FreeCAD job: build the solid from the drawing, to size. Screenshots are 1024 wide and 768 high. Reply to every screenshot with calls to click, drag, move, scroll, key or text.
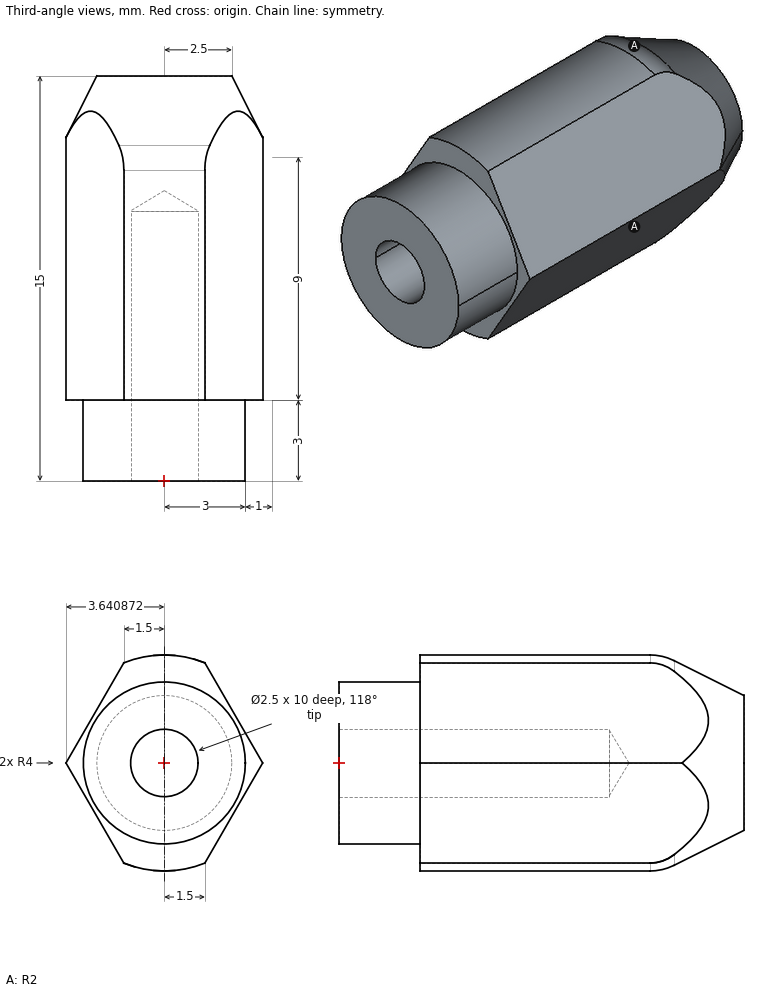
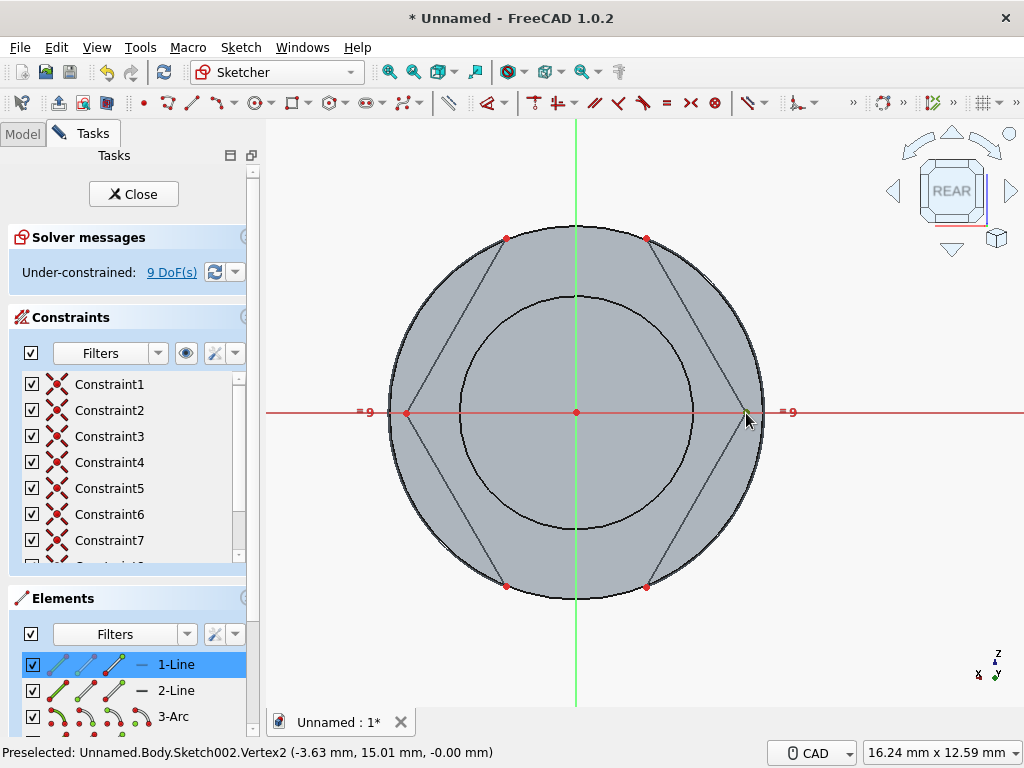
click(406, 414)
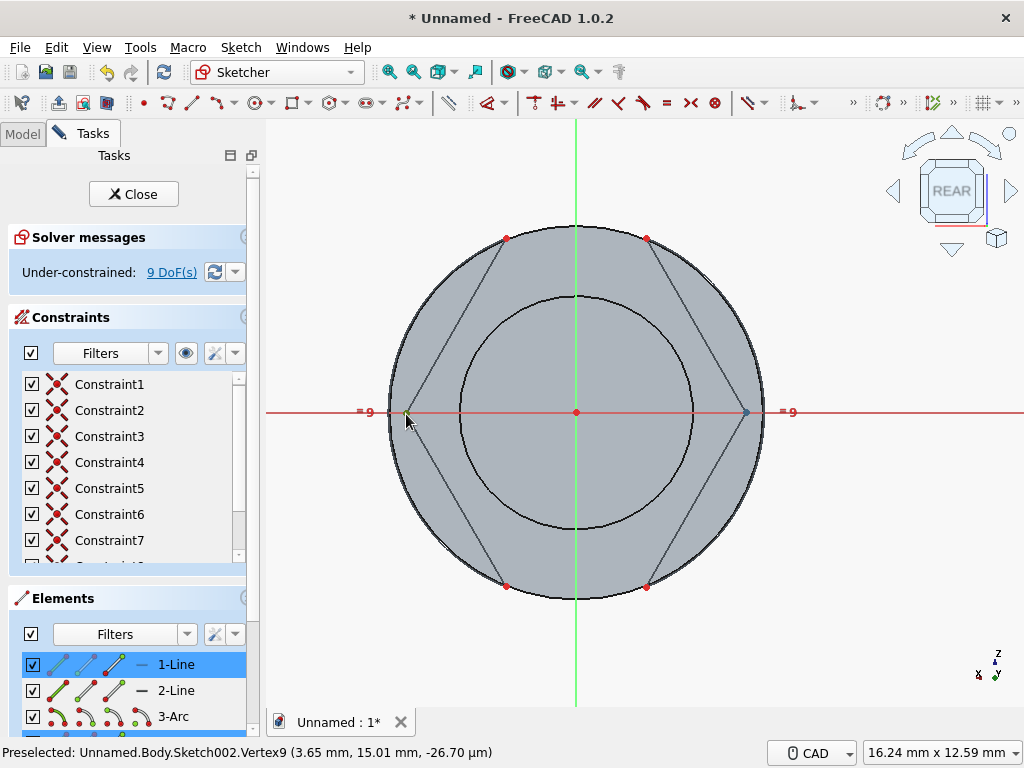
click(576, 641)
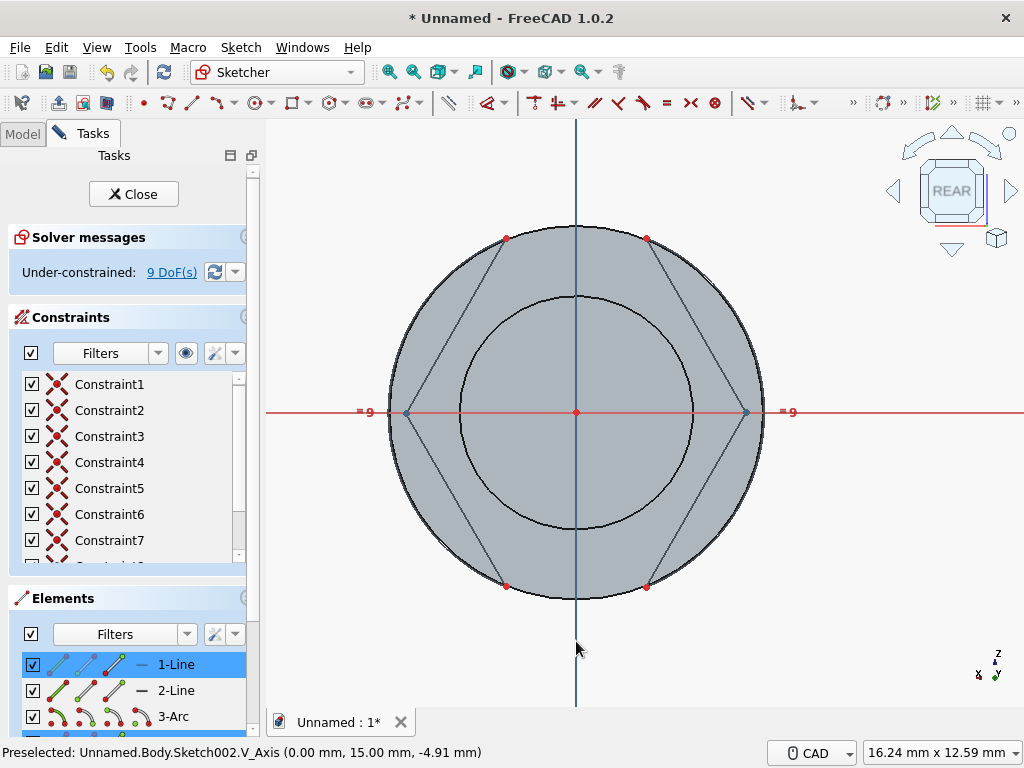
click(692, 104)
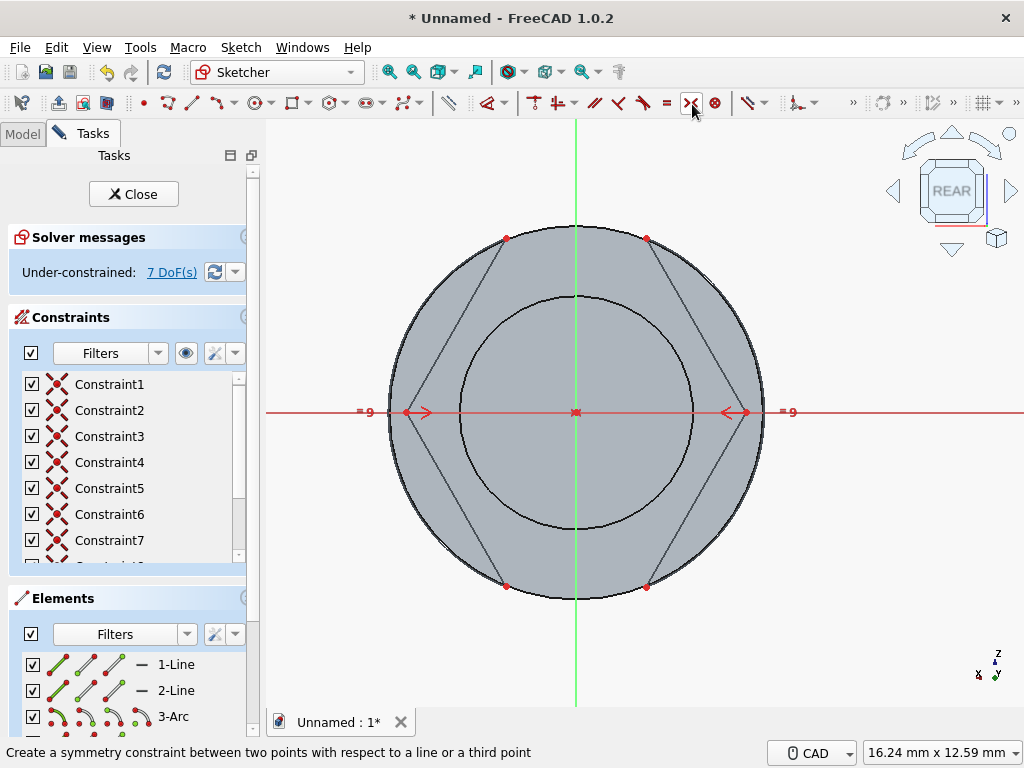
click(488, 104)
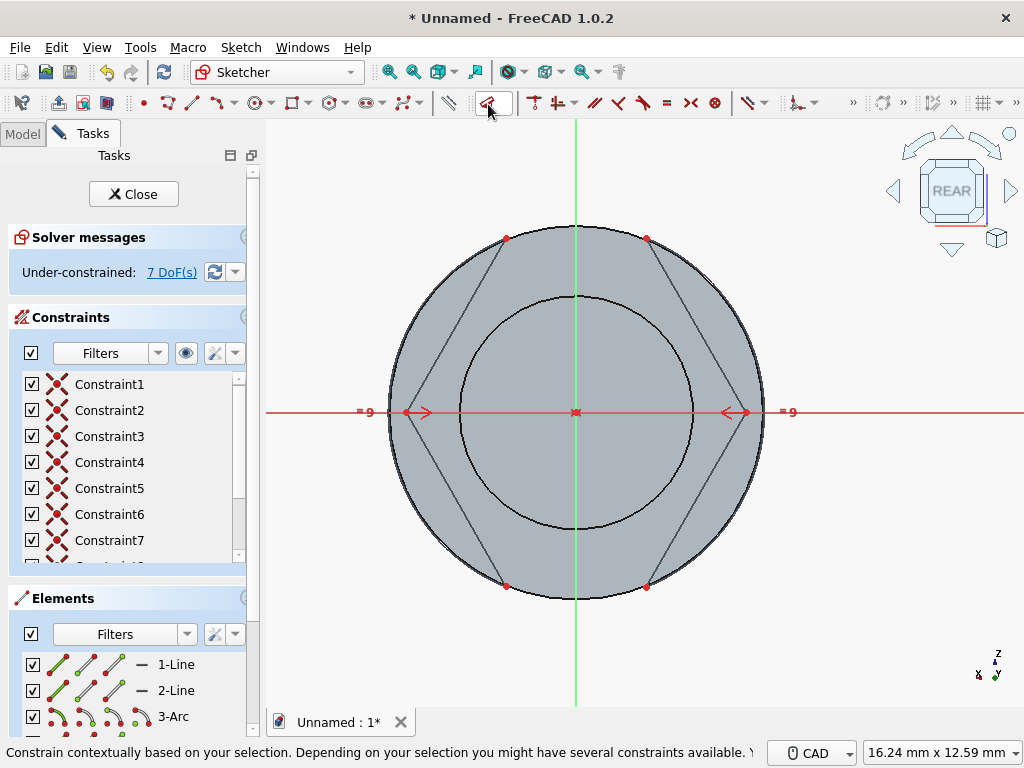
click(743, 499)
click(771, 514)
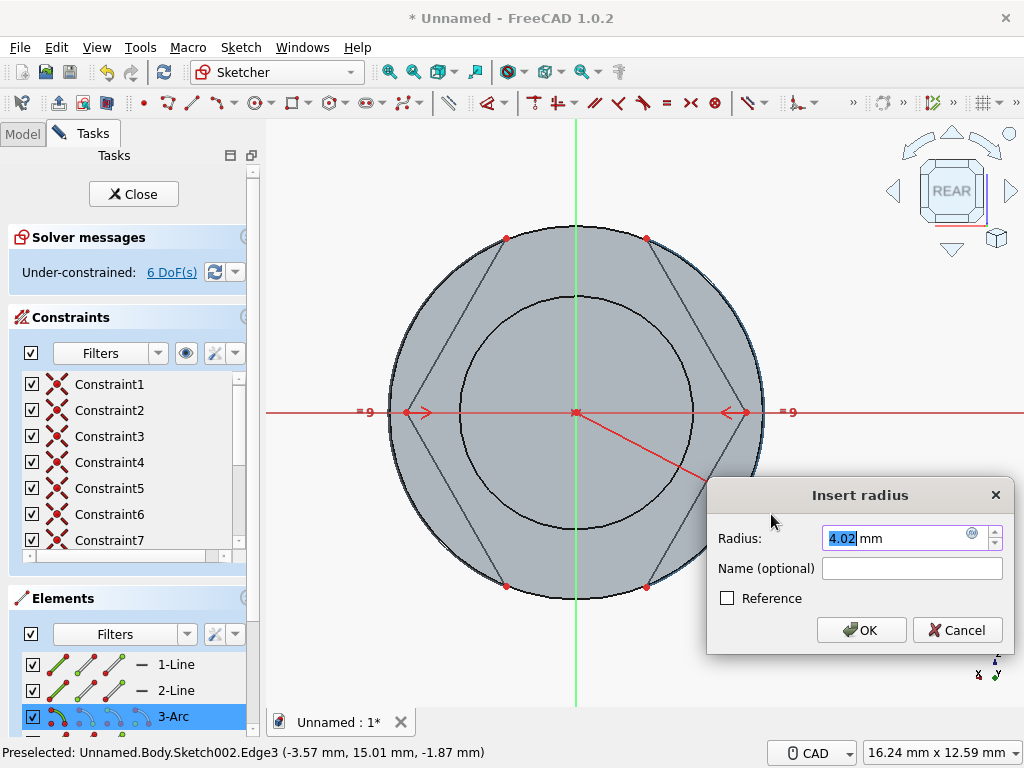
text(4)
key(Return)
key(Escape)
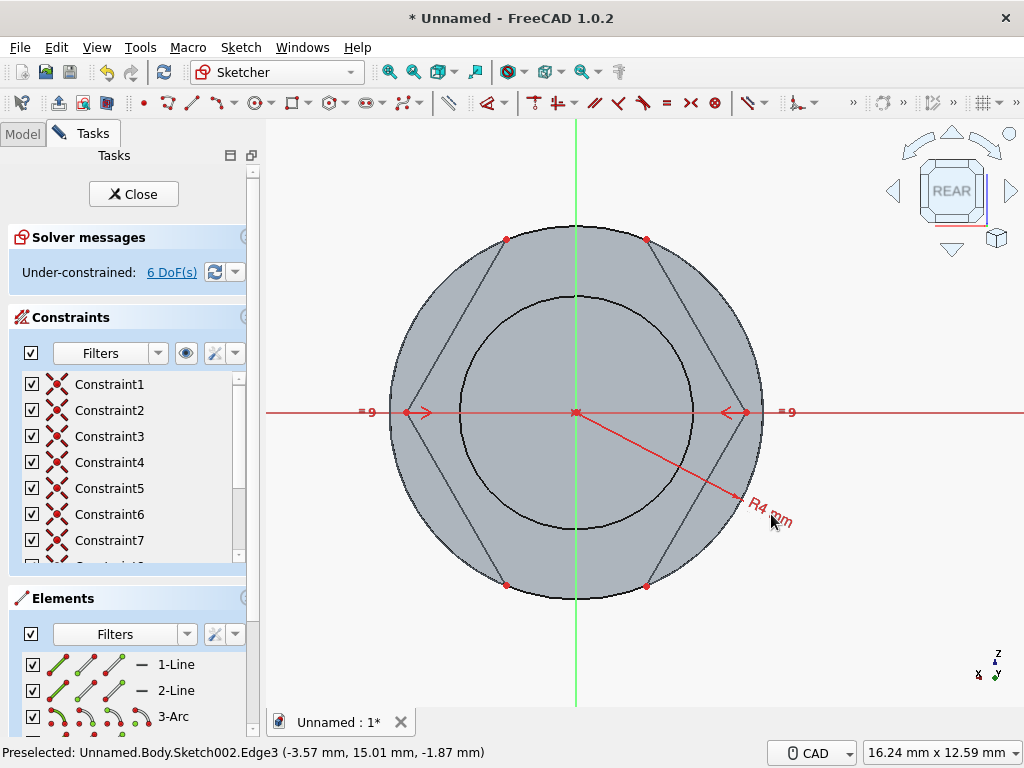
click(746, 413)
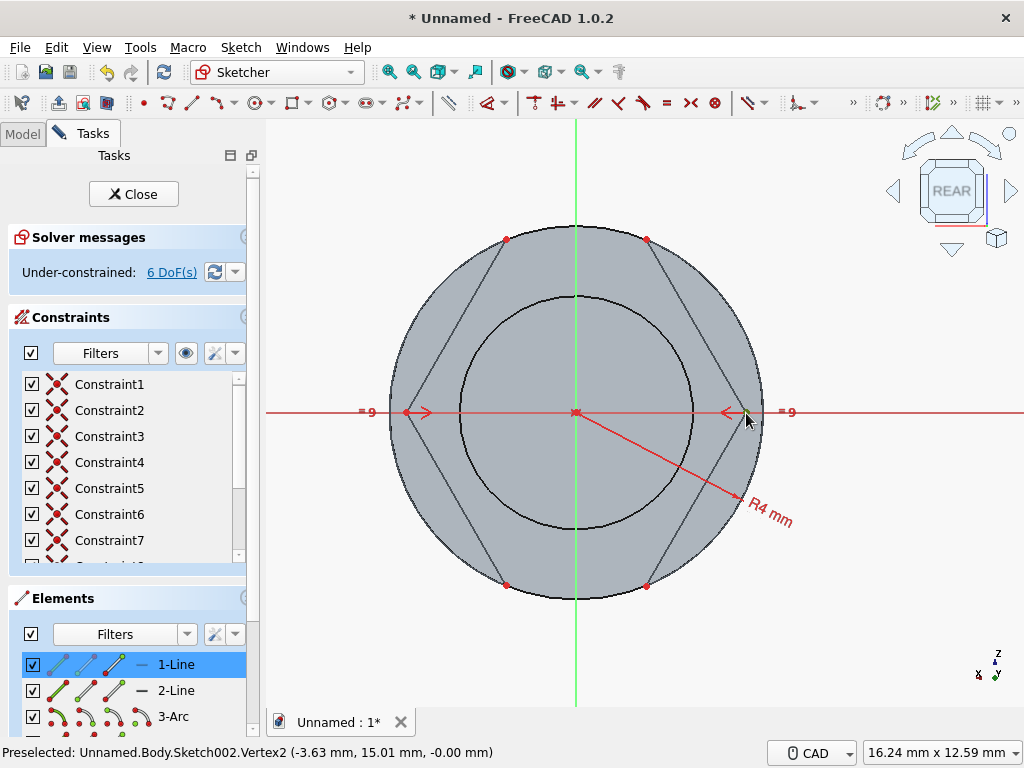
click(334, 413)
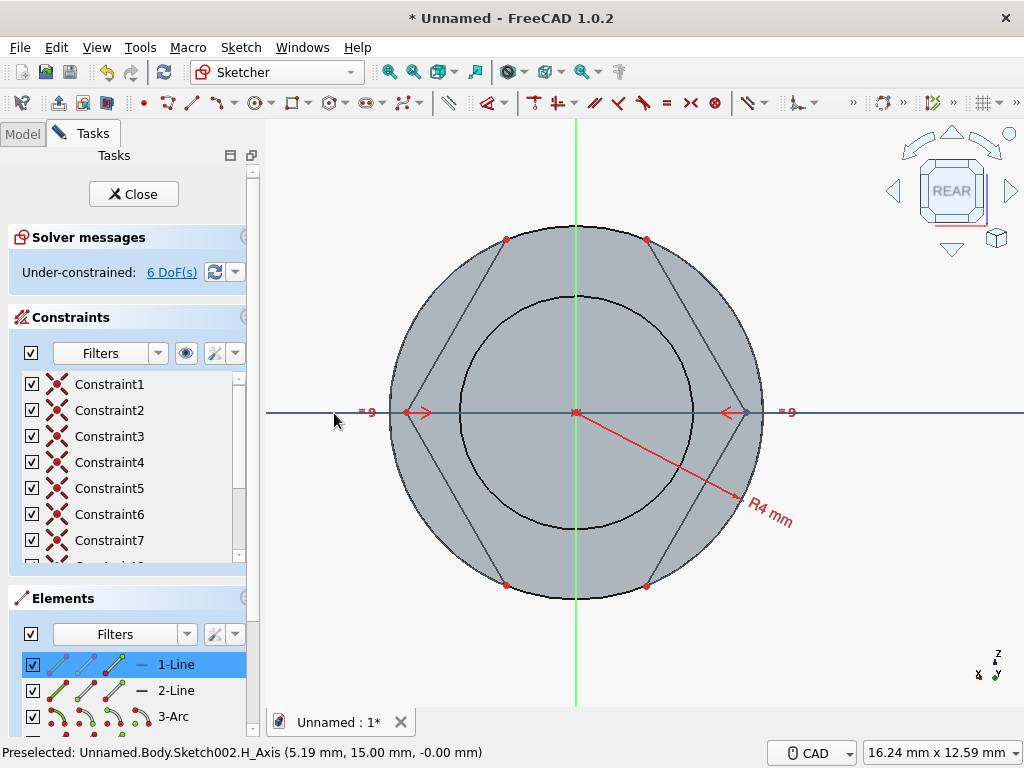
click(534, 104)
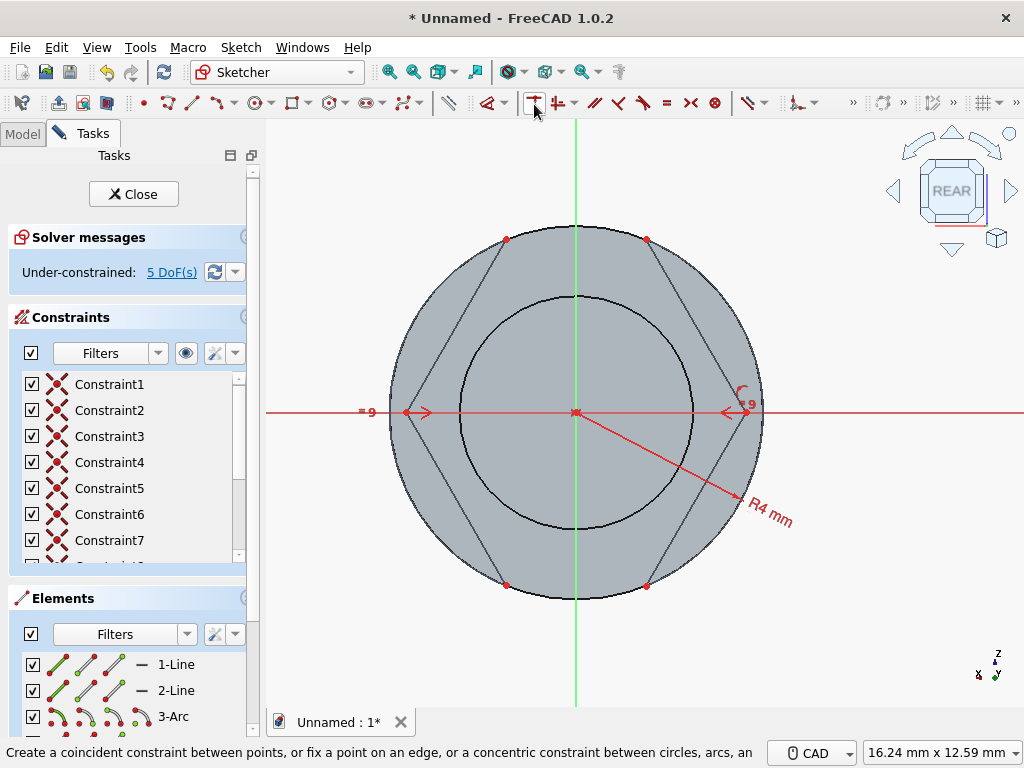
click(488, 104)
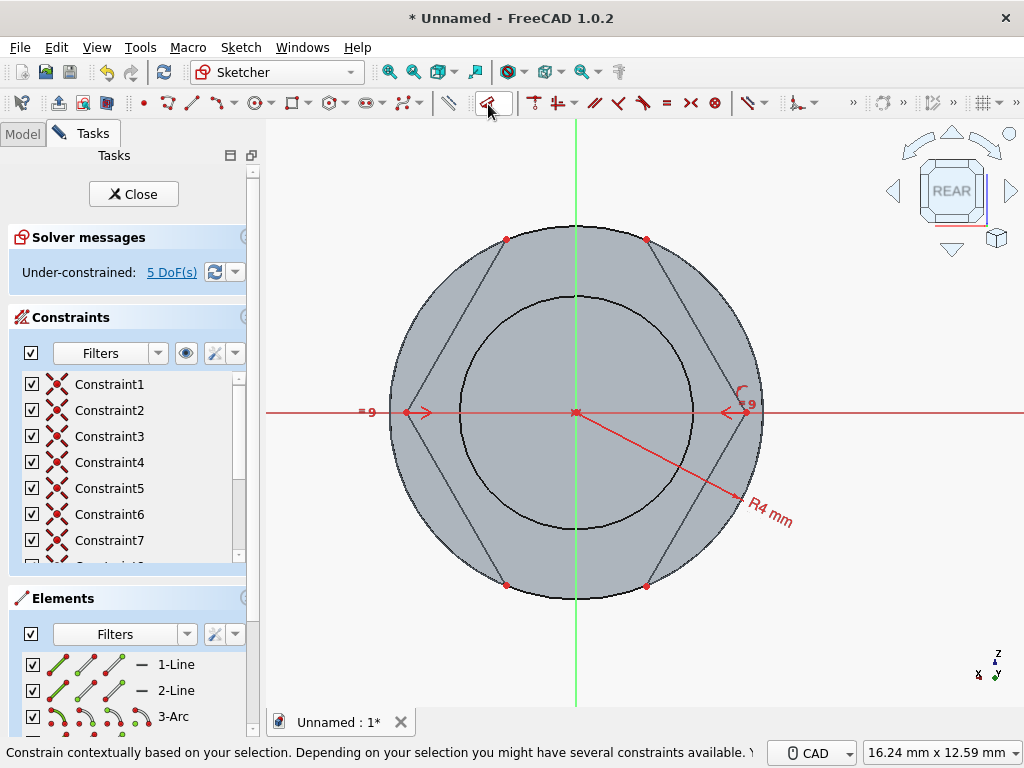
click(646, 239)
click(611, 205)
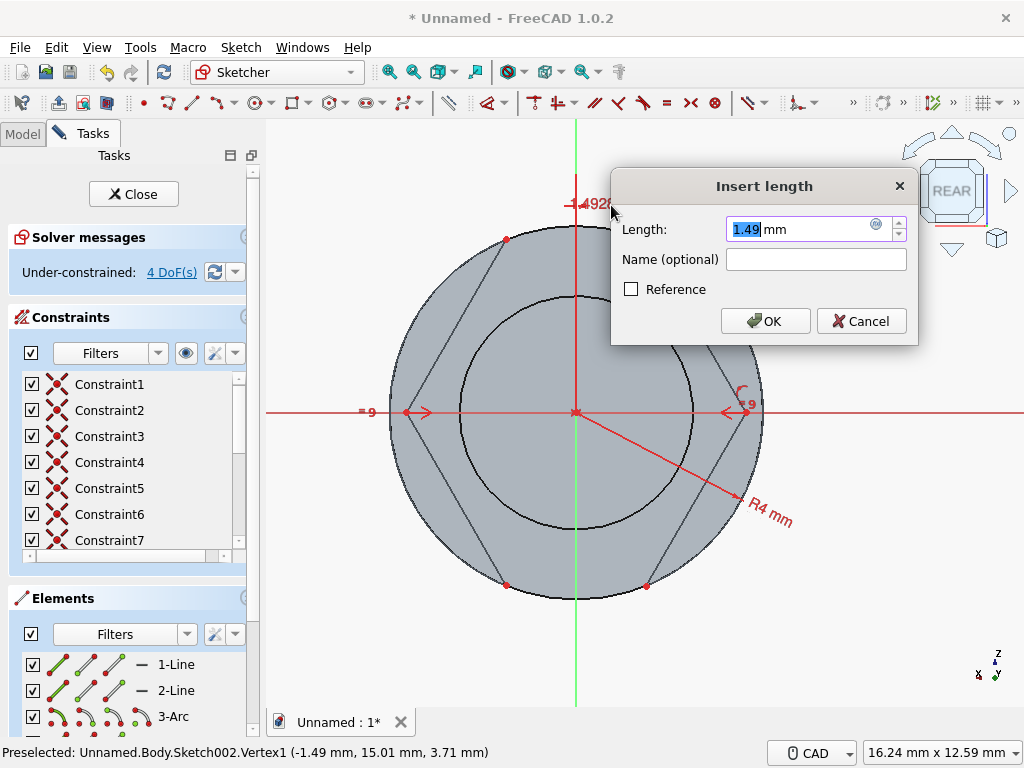
text(1.5)
key(Return)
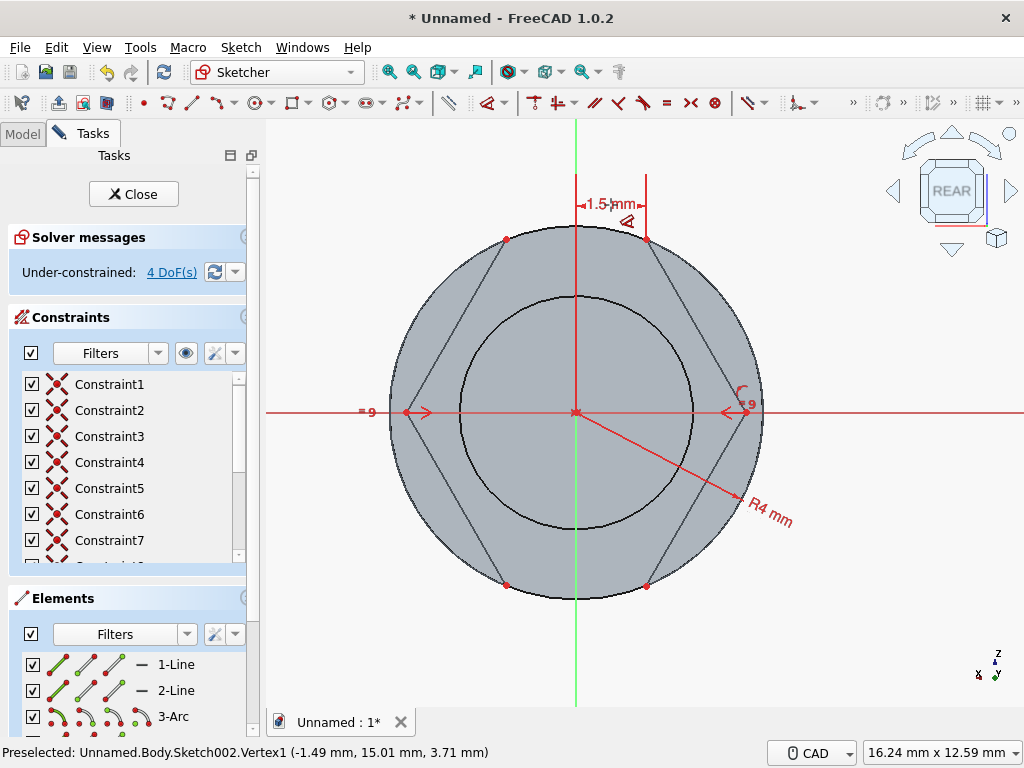
click(646, 586)
click(611, 620)